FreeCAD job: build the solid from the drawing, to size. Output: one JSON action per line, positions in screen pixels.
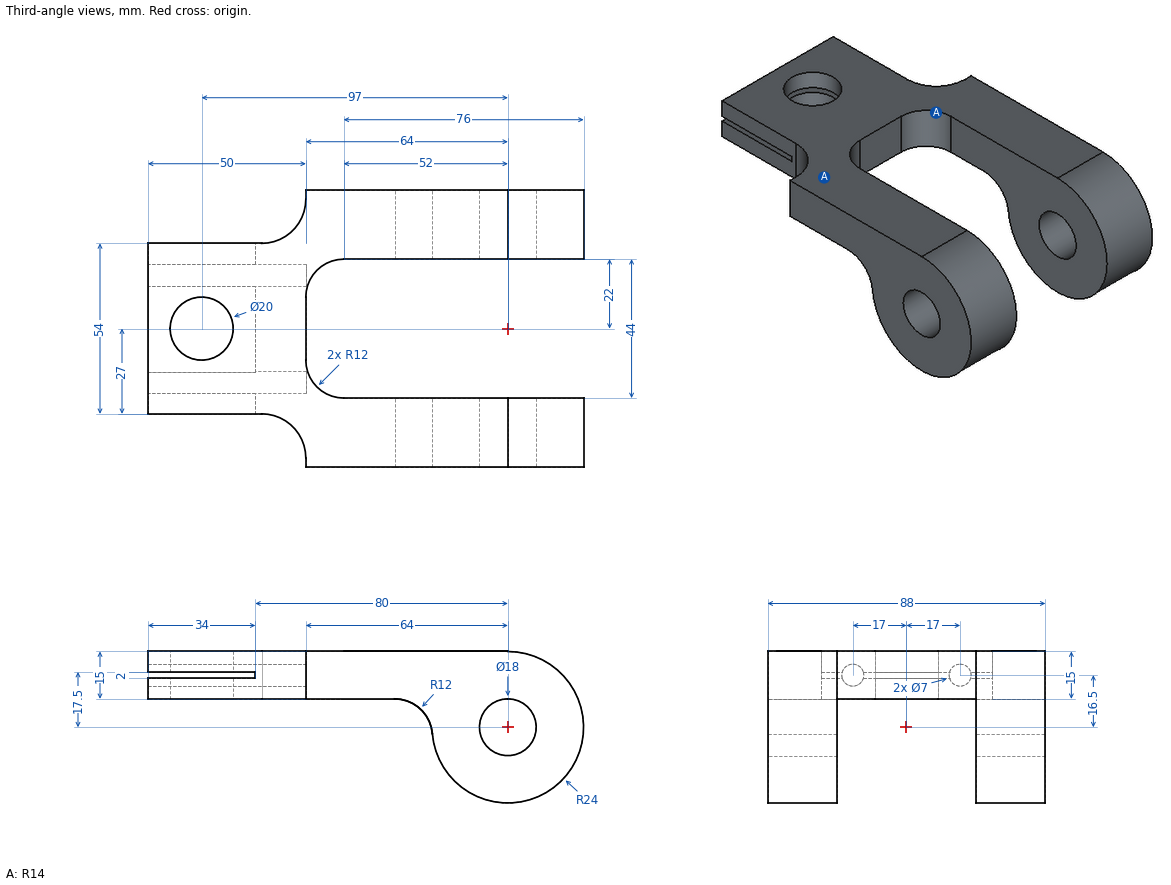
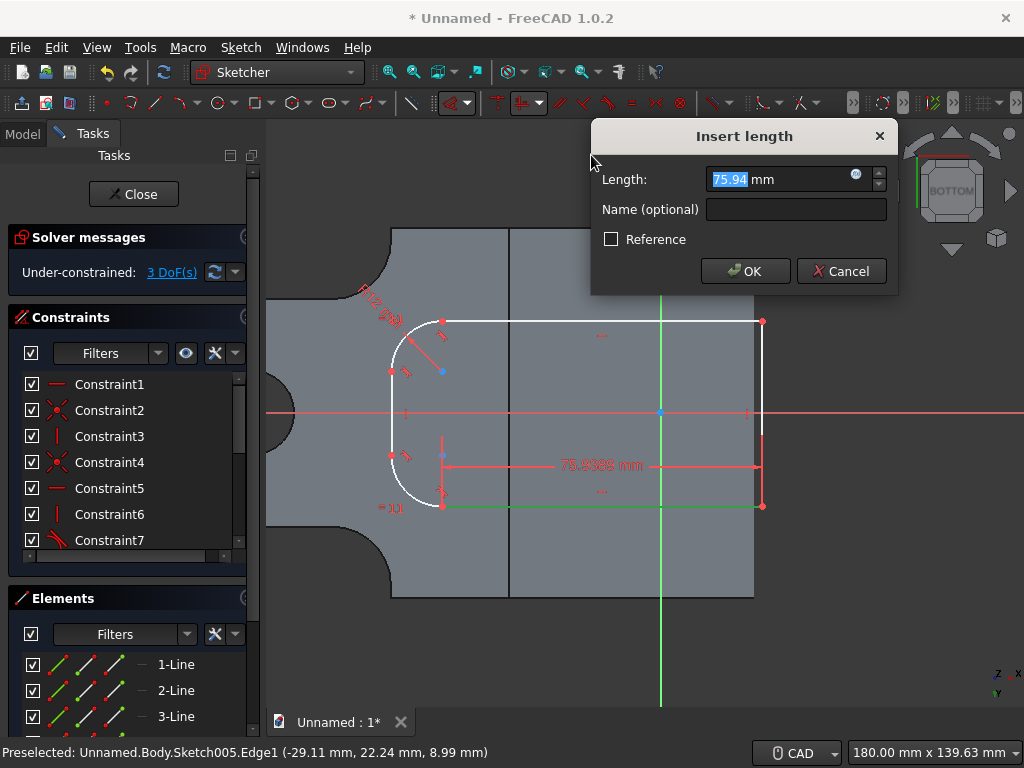
{"action": "type", "text": "76"}
{"action": "key", "text": "Return"}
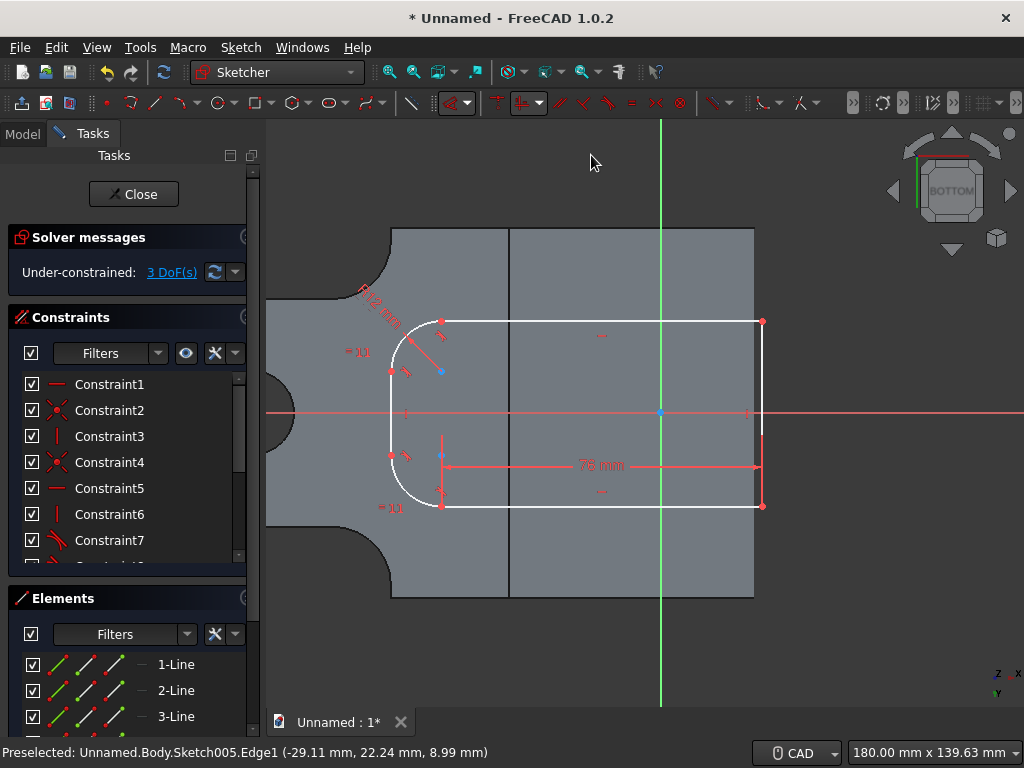
{"action": "left_click", "coordinate": [762, 451]}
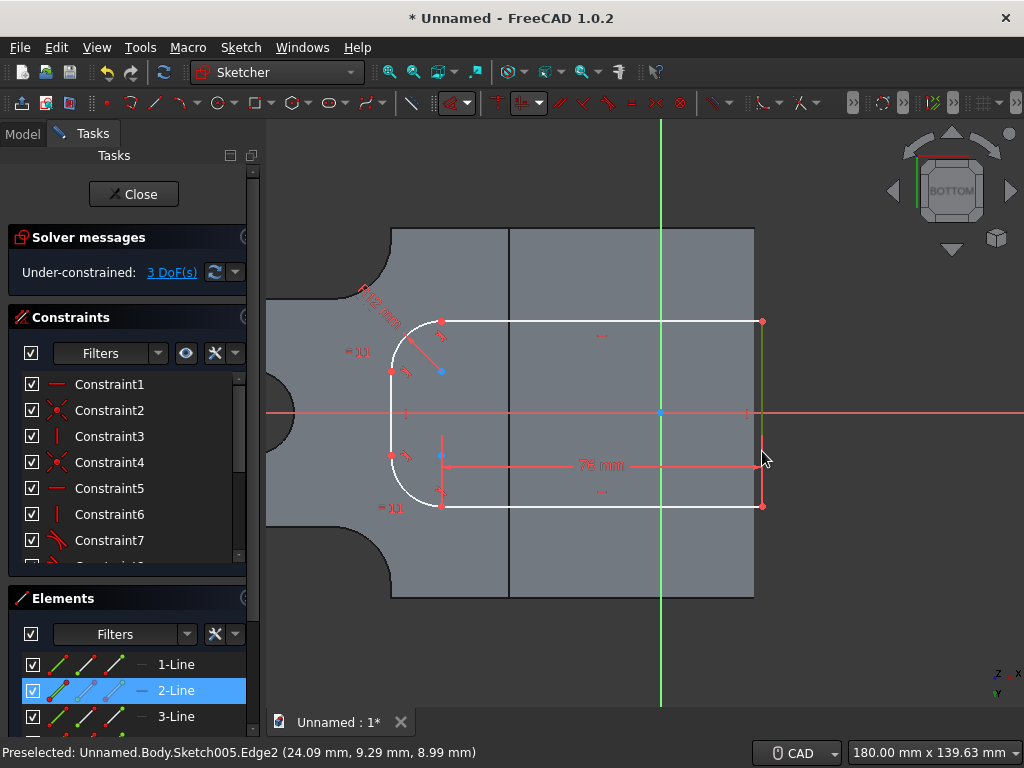
{"action": "left_click", "coordinate": [470, 104]}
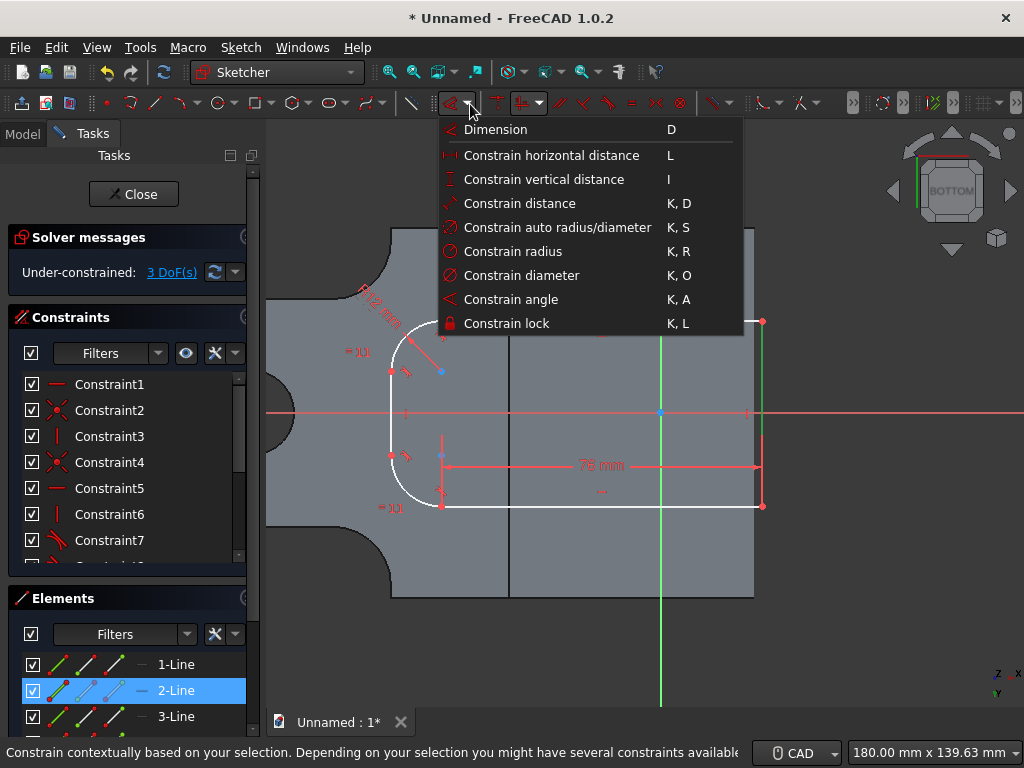
{"action": "left_click", "coordinate": [591, 179]}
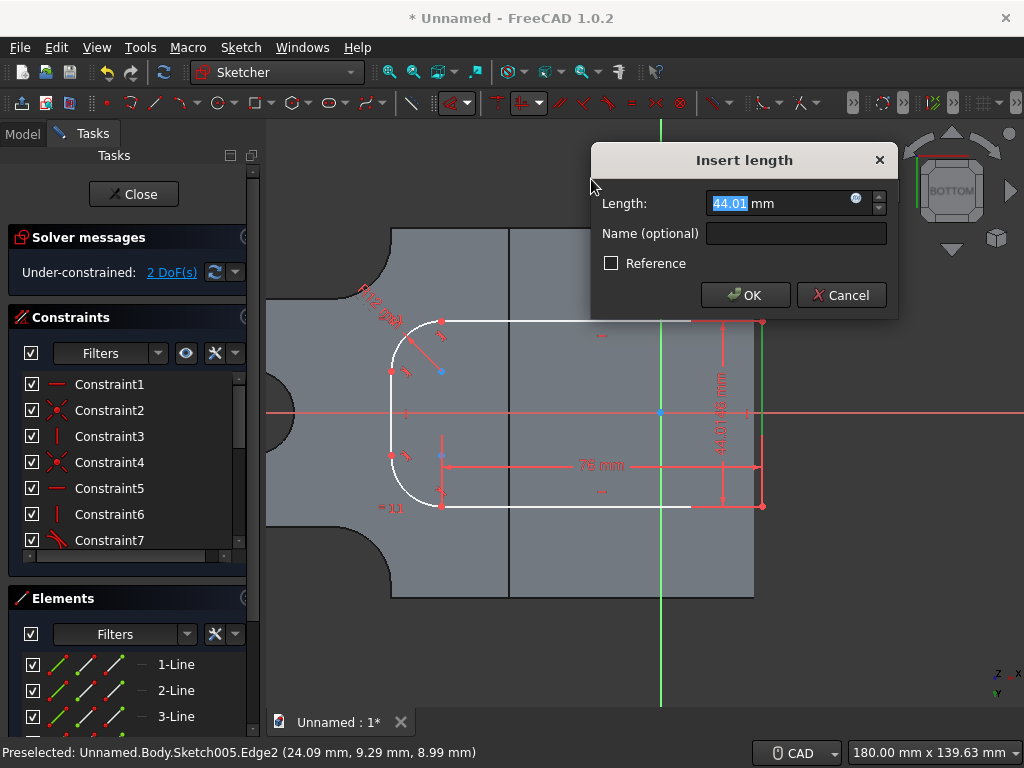
{"action": "type", "text": "44"}
{"action": "key", "text": "Return"}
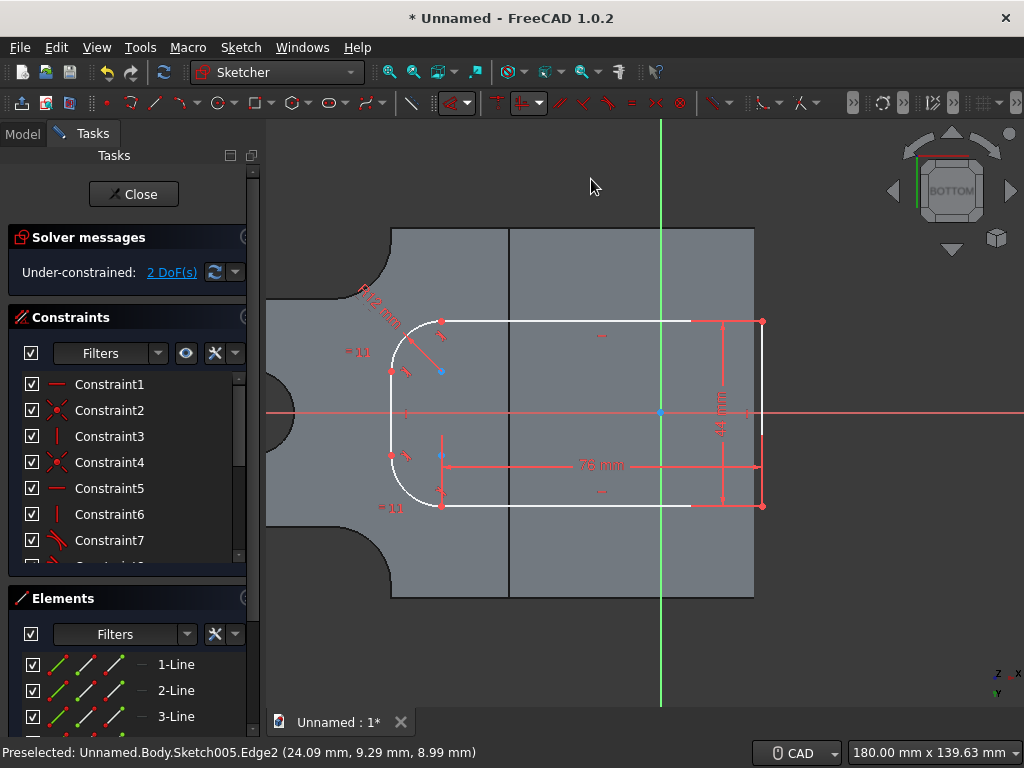
{"action": "left_click", "coordinate": [442, 506]}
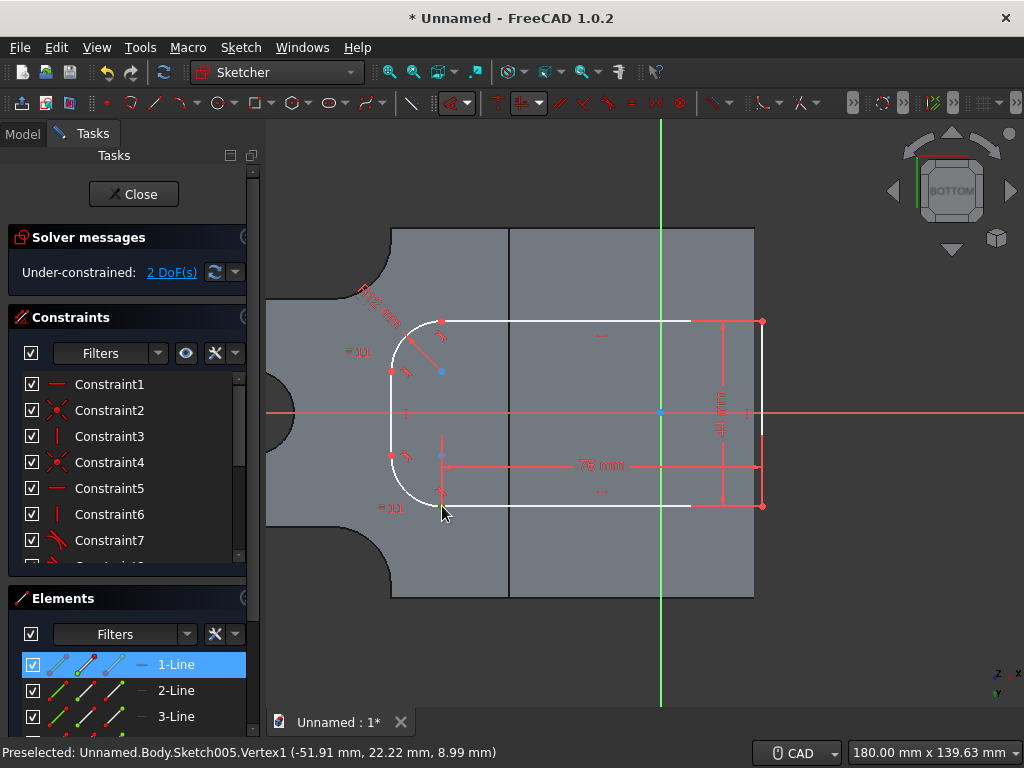
{"action": "key", "text": "l"}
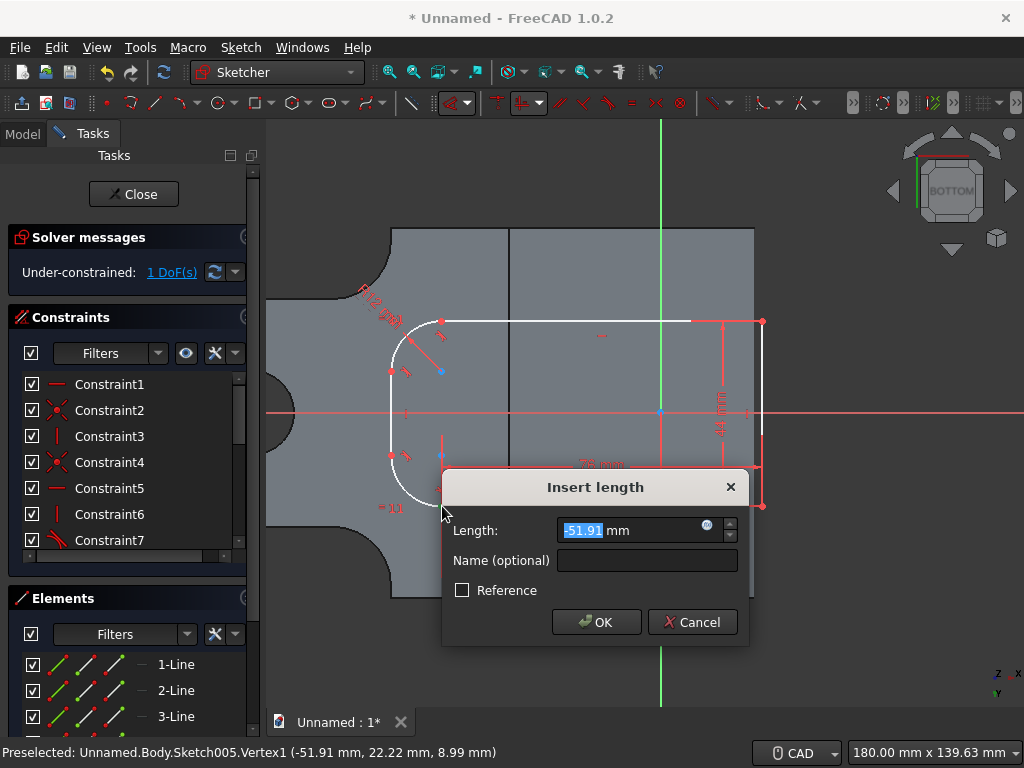
{"action": "type", "text": "-52"}
{"action": "key", "text": "Return"}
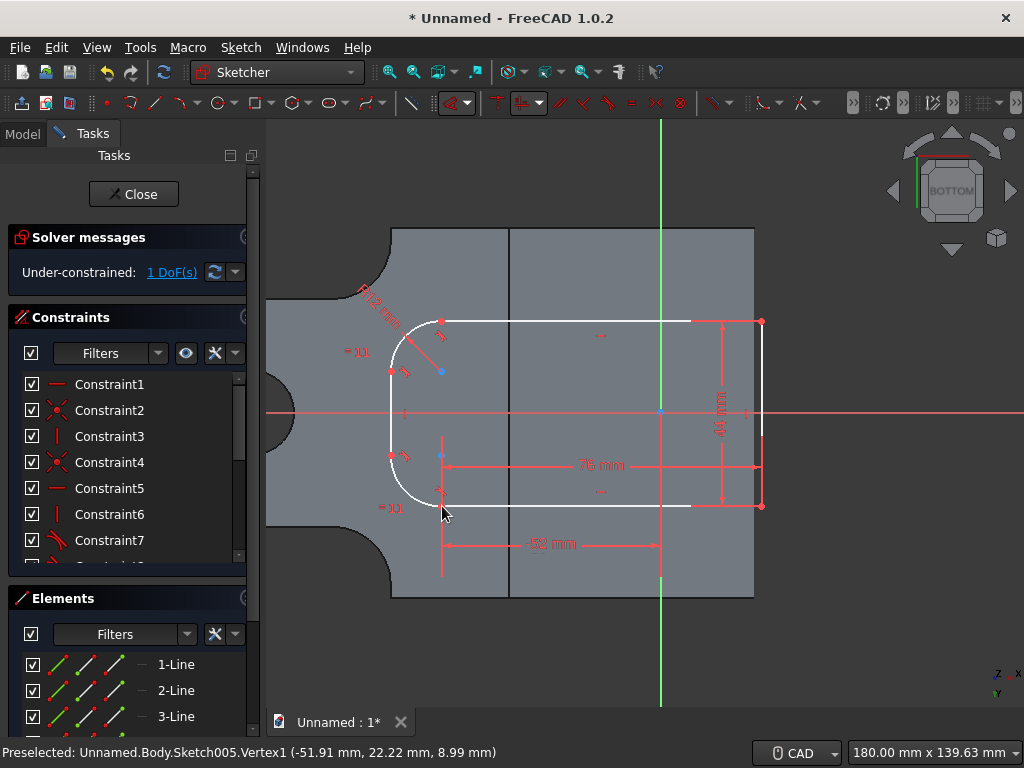
{"action": "left_click", "coordinate": [442, 506]}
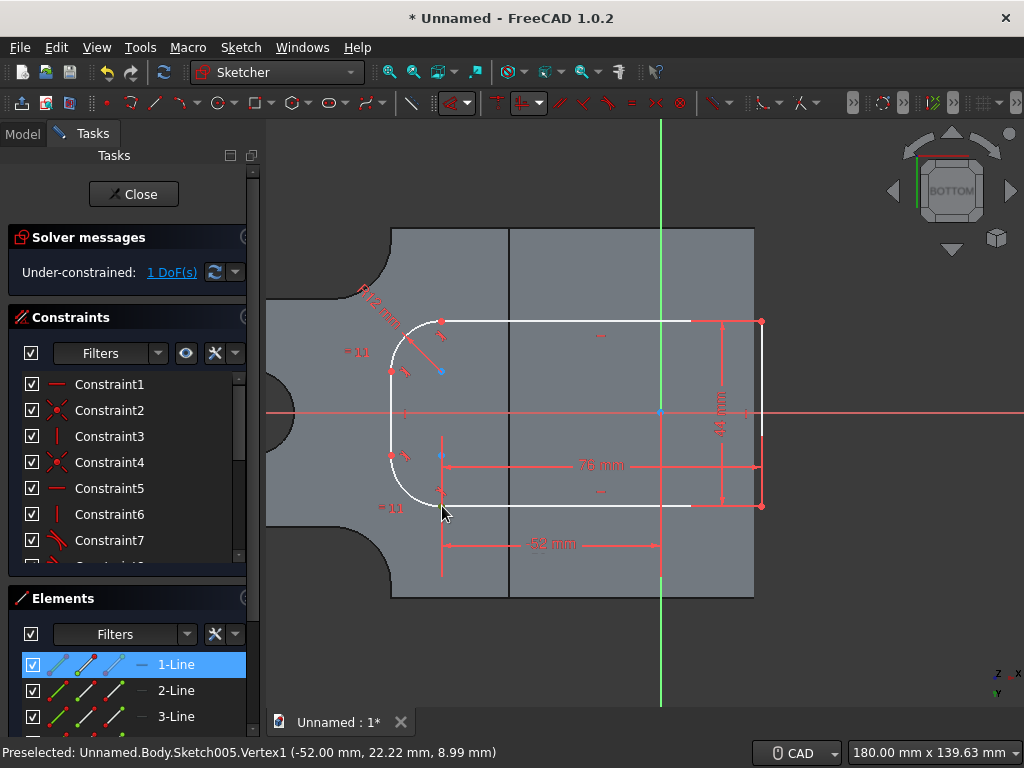
{"action": "left_click", "coordinate": [470, 104]}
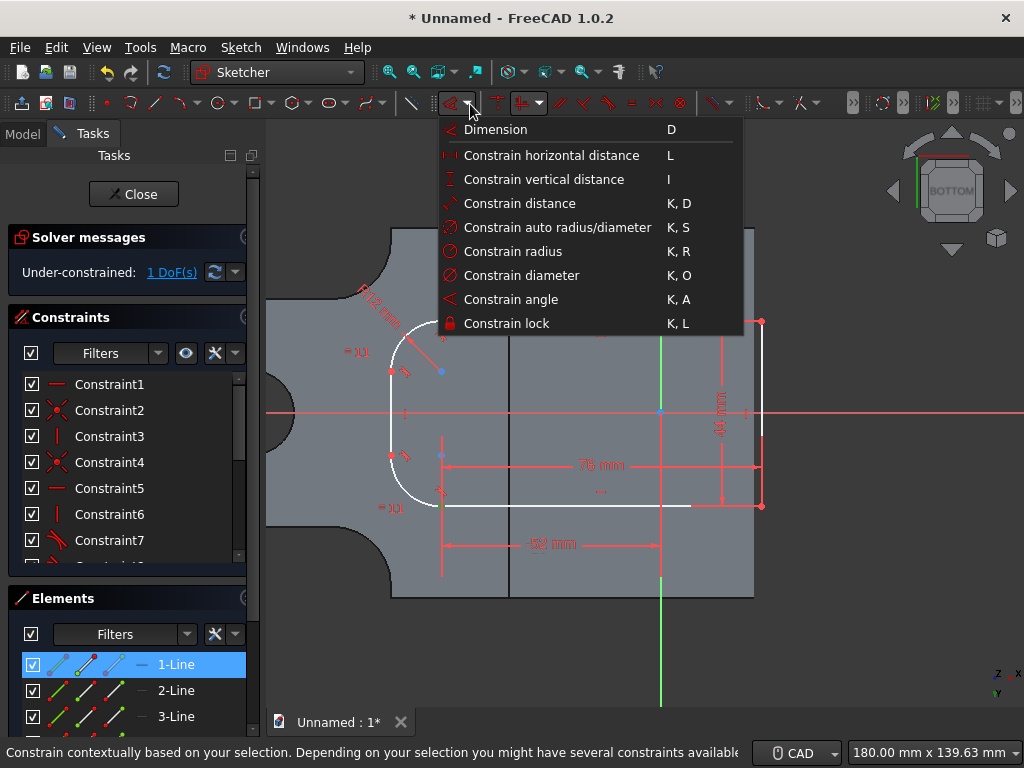
{"action": "left_click", "coordinate": [591, 179]}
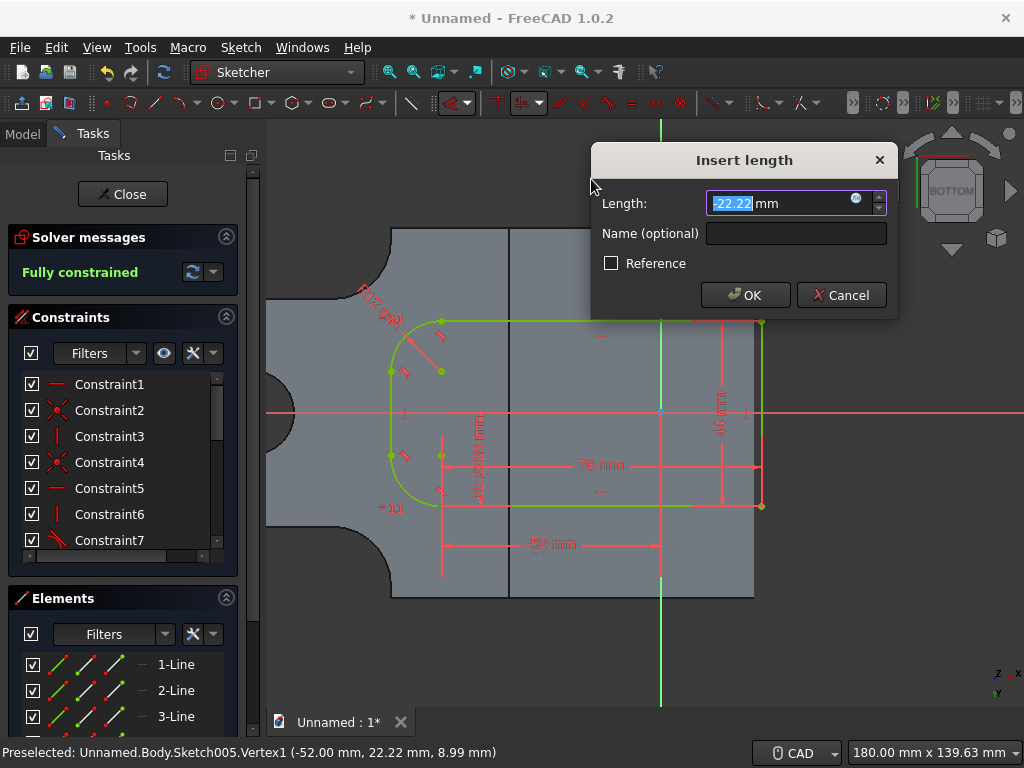
{"action": "type", "text": "-22"}
{"action": "key", "text": "Return"}